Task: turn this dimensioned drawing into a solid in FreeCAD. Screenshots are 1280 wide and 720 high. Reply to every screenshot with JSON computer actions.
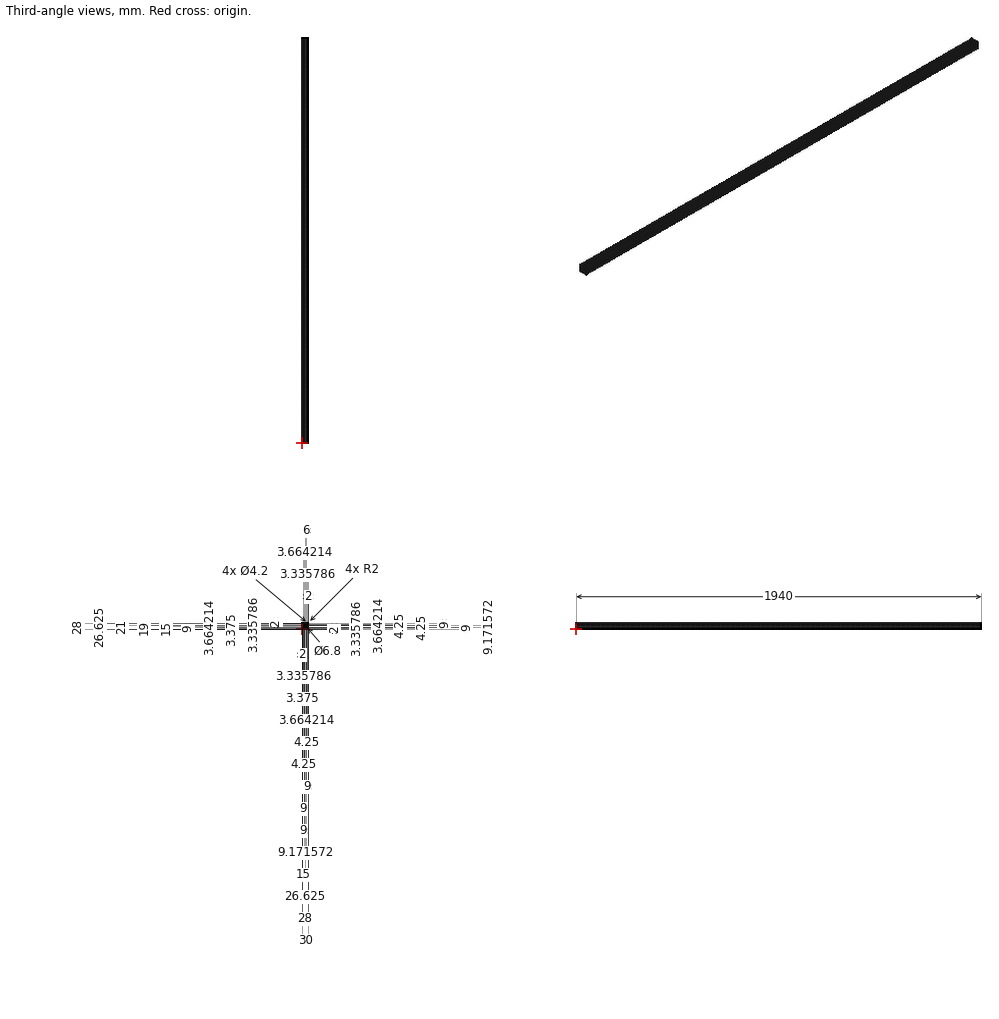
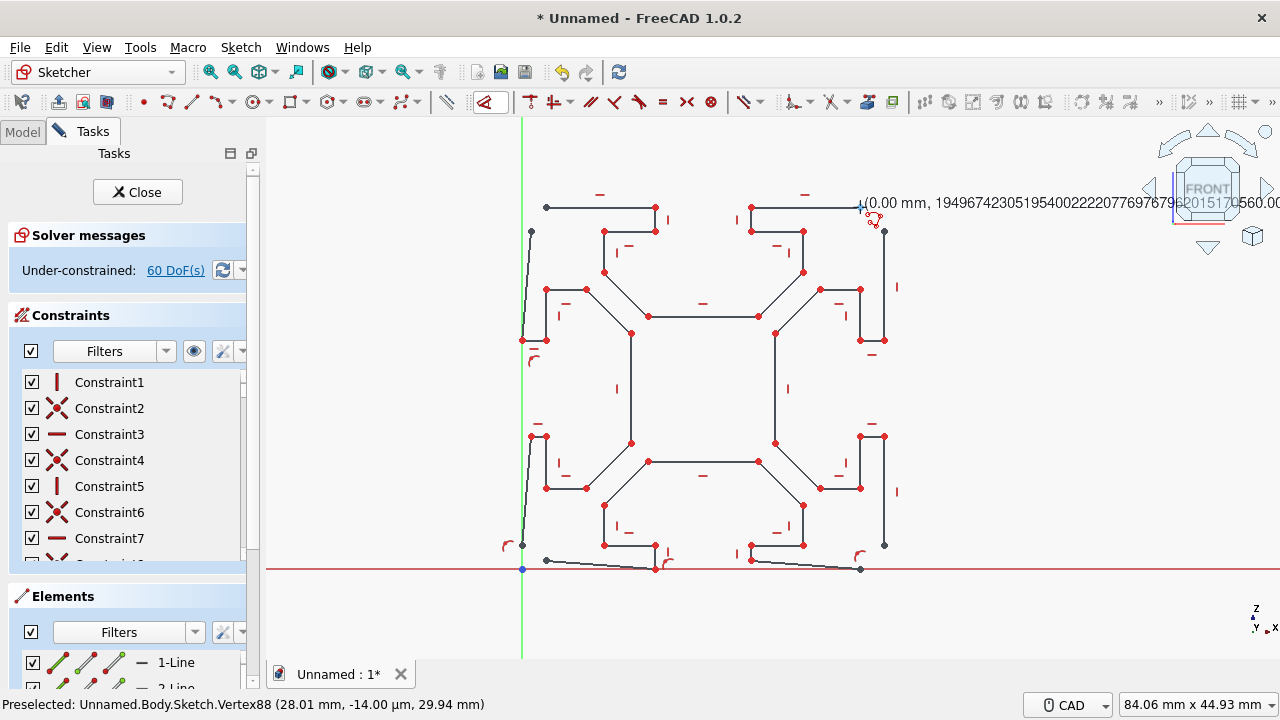
{"action": "left_click", "coordinate": [216, 102]}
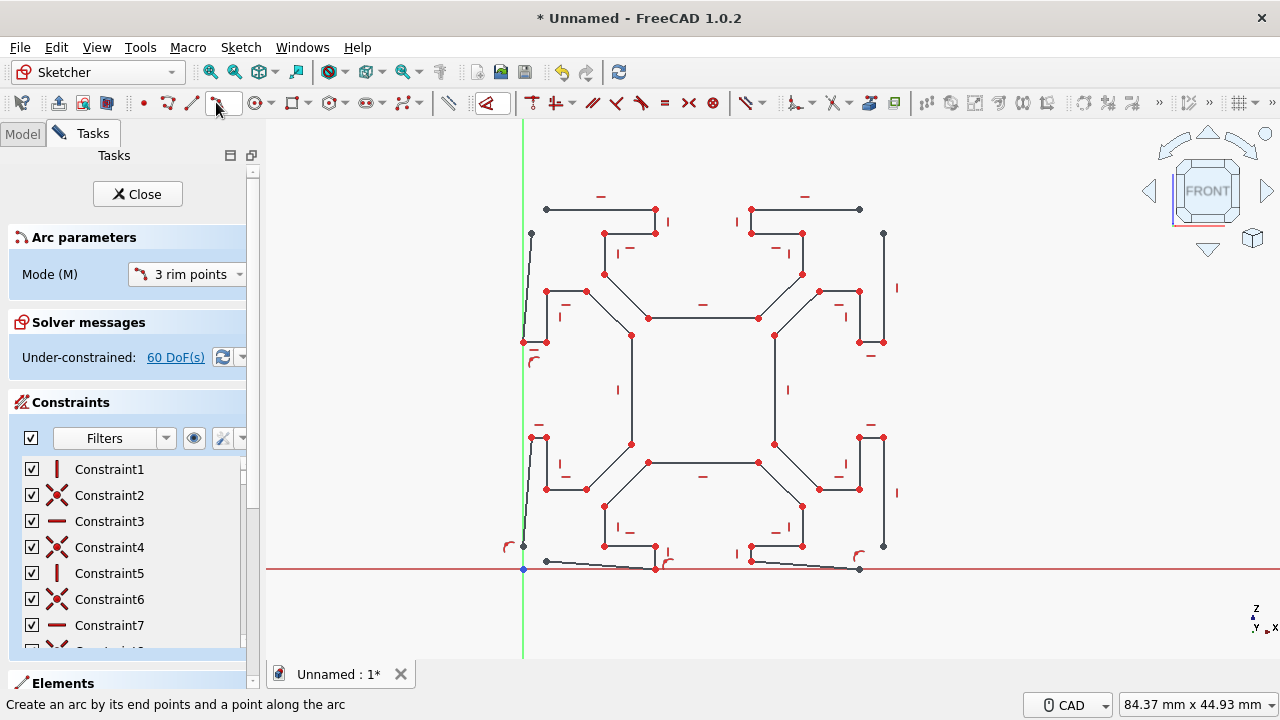
{"action": "left_click", "coordinate": [884, 546]}
{"action": "left_click", "coordinate": [860, 569]}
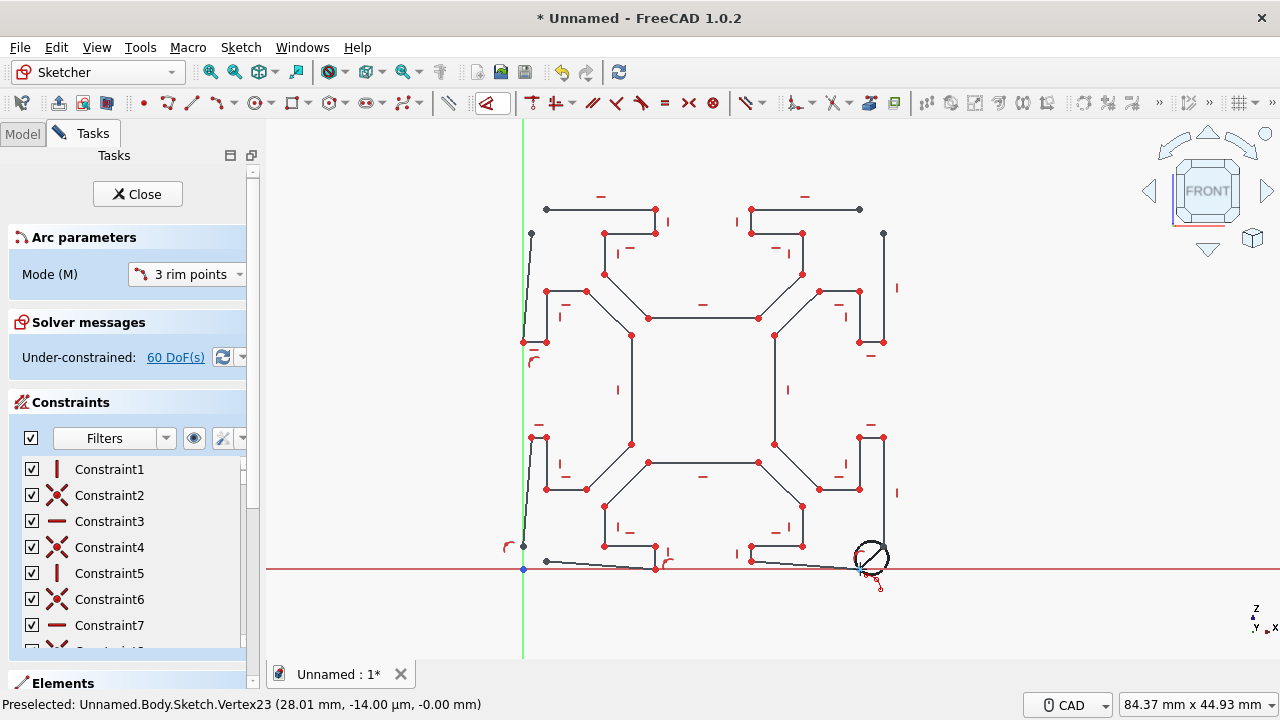
{"action": "scroll", "coordinate": [877, 562], "scroll_direction": "up", "scroll_amount": 5}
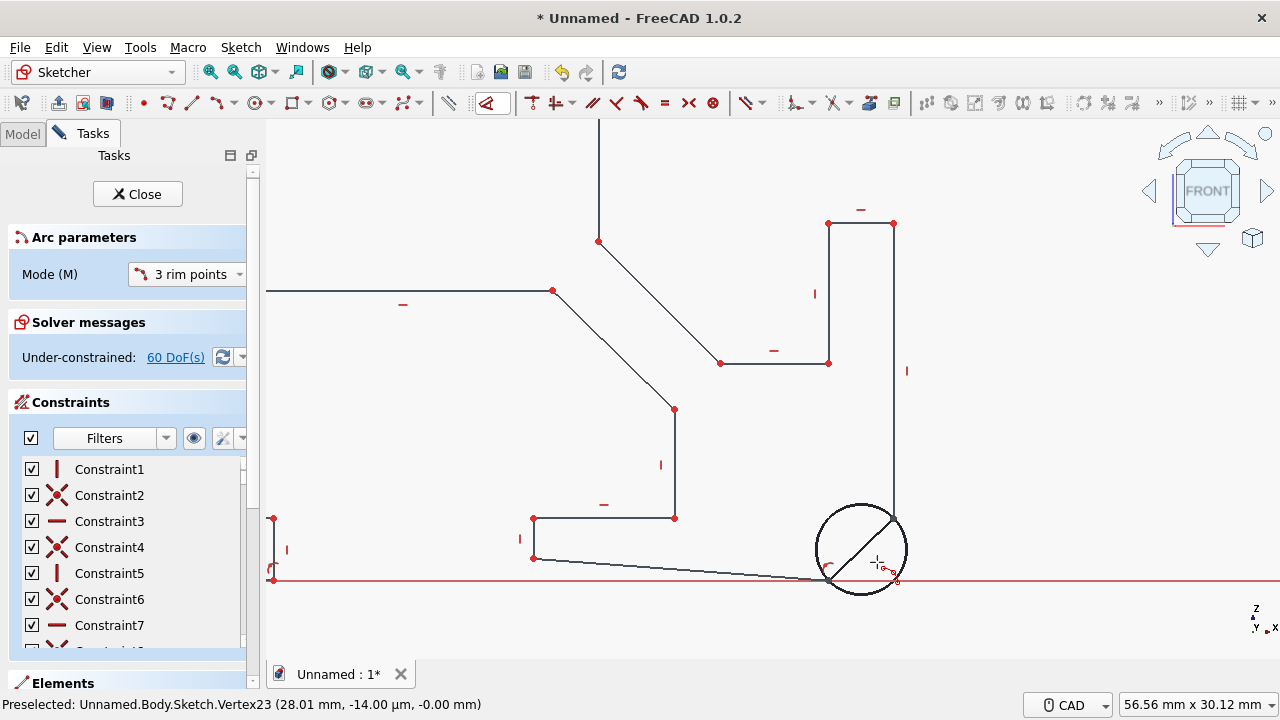
{"action": "left_click", "coordinate": [875, 562]}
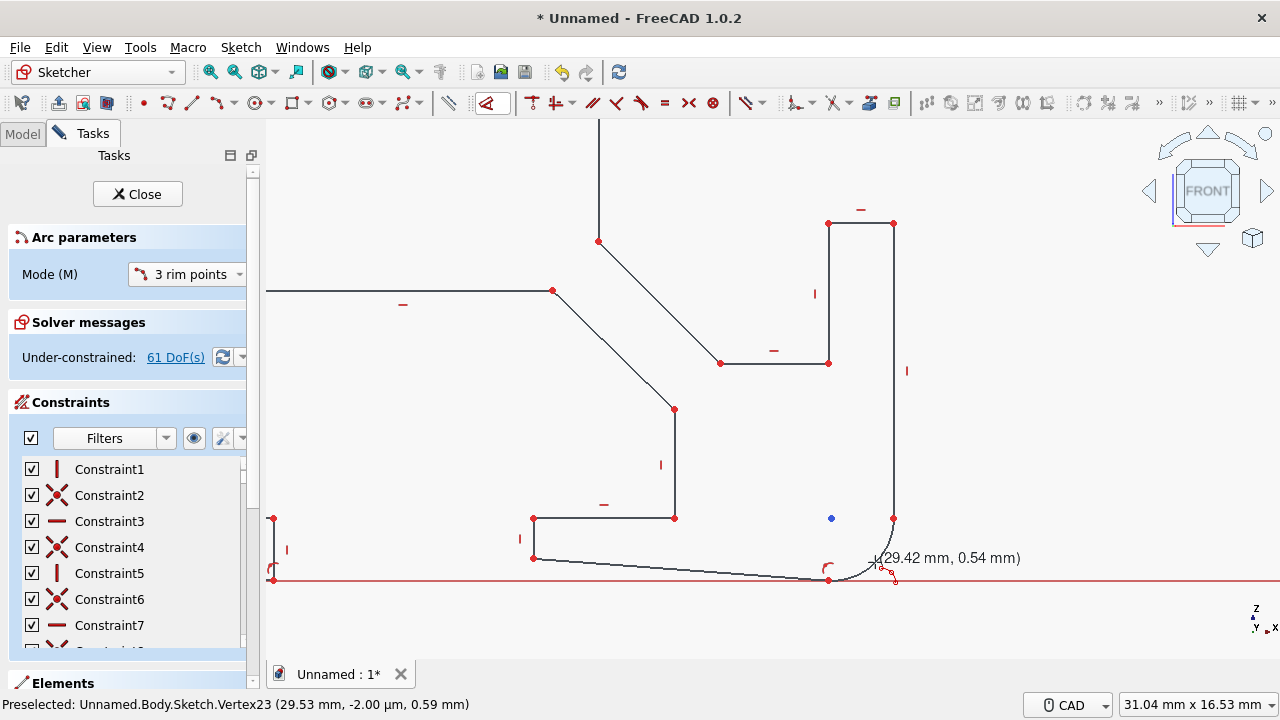
{"action": "scroll", "coordinate": [879, 563], "scroll_direction": "down", "scroll_amount": 5}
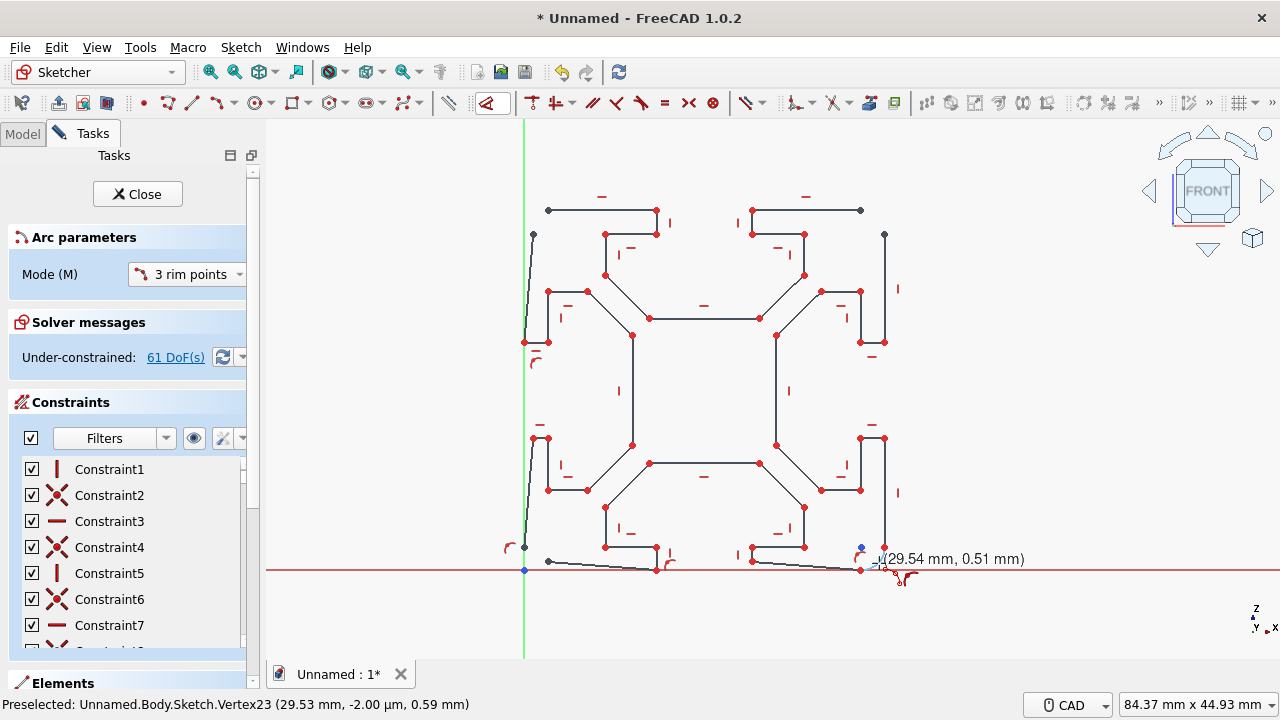
{"action": "left_click", "coordinate": [548, 562]}
{"action": "left_click", "coordinate": [524, 547]}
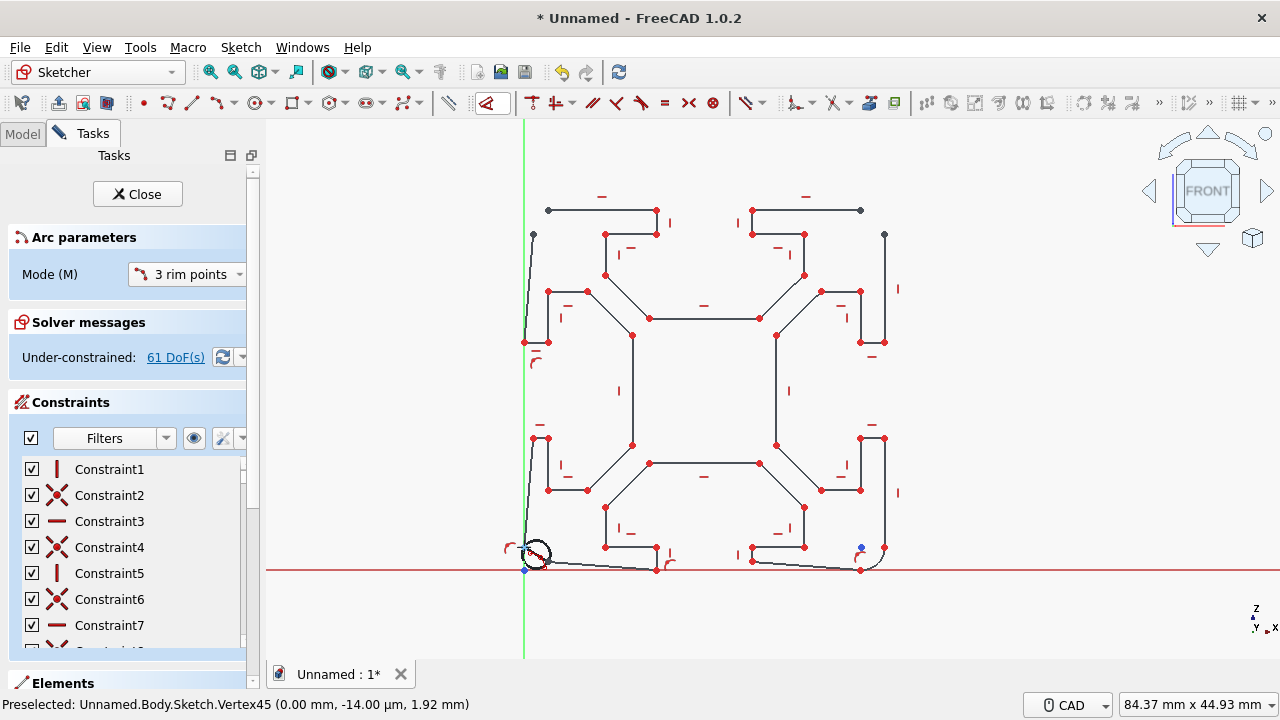
{"action": "scroll", "coordinate": [531, 563], "scroll_direction": "up", "scroll_amount": 5}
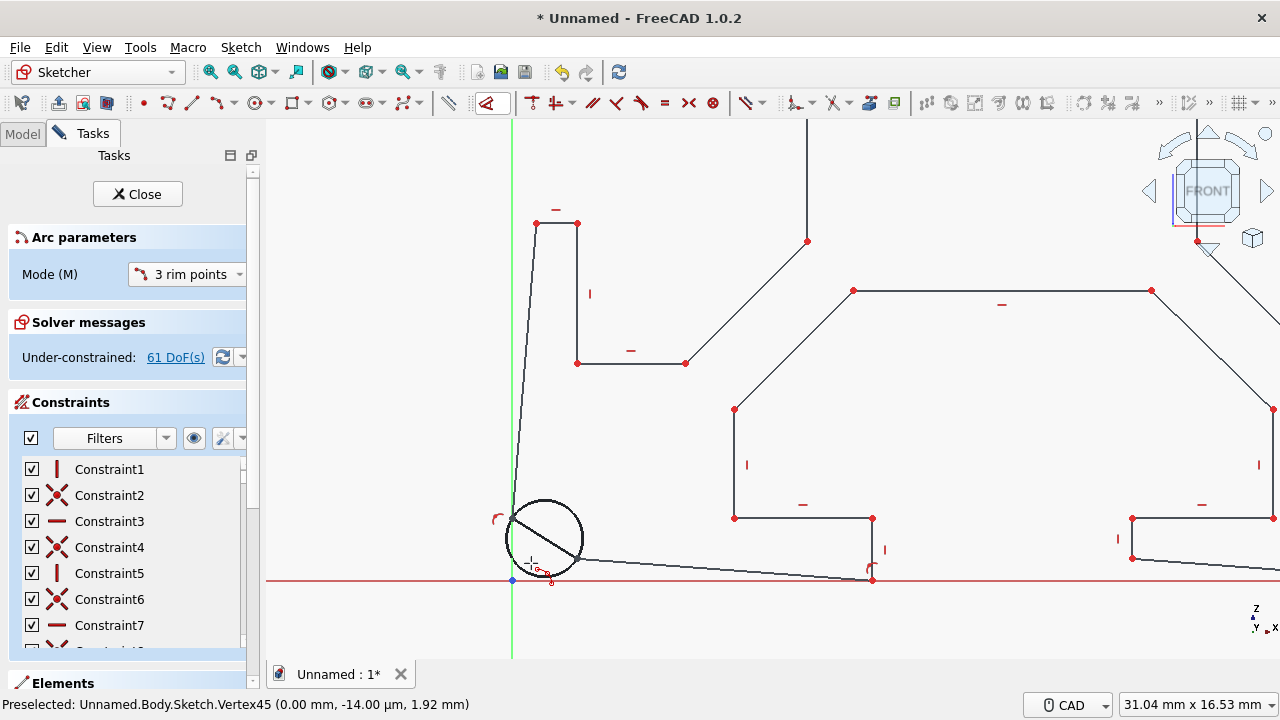
{"action": "left_click", "coordinate": [532, 562]}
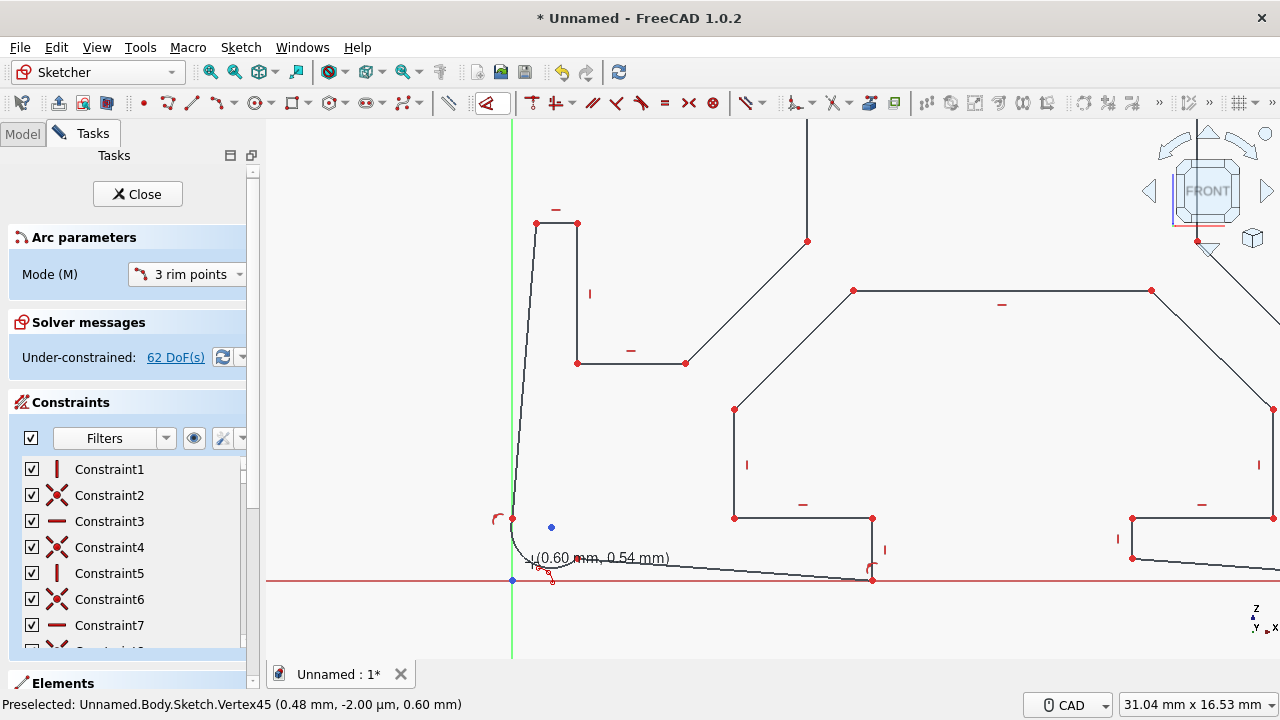
{"action": "scroll", "coordinate": [531, 563], "scroll_direction": "down", "scroll_amount": 5}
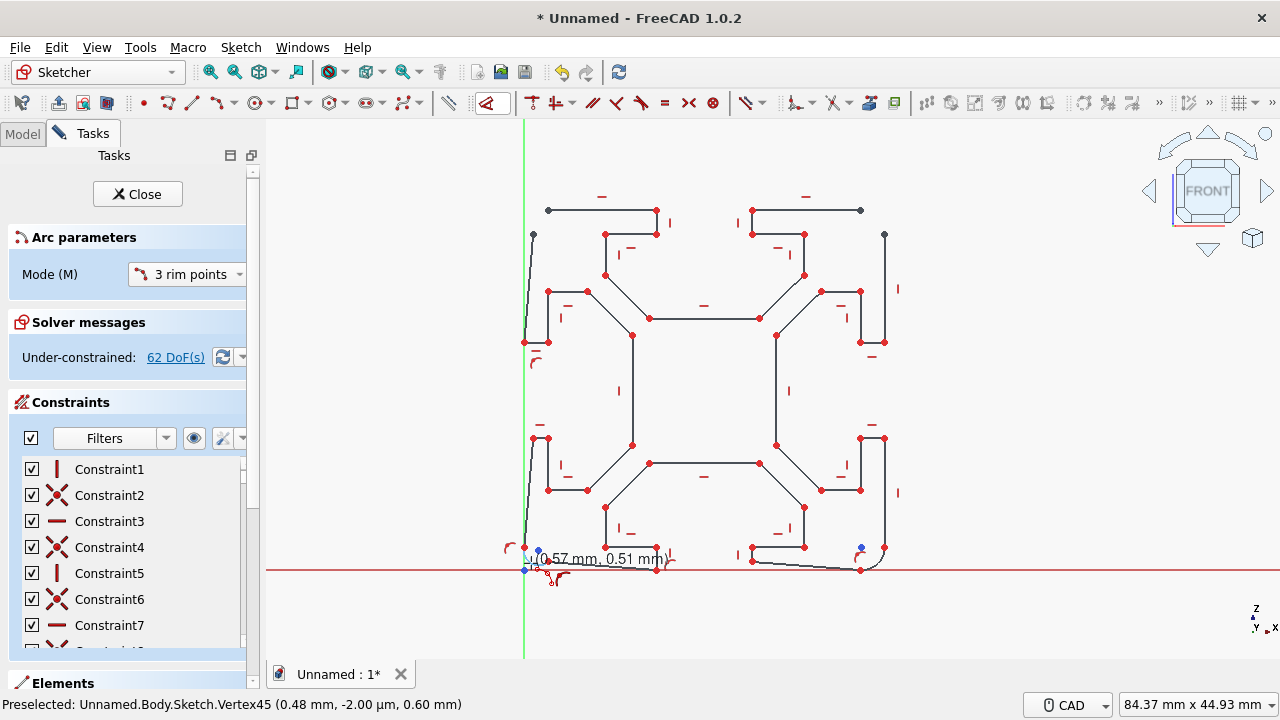
{"action": "left_click", "coordinate": [533, 234]}
{"action": "left_click", "coordinate": [548, 210]}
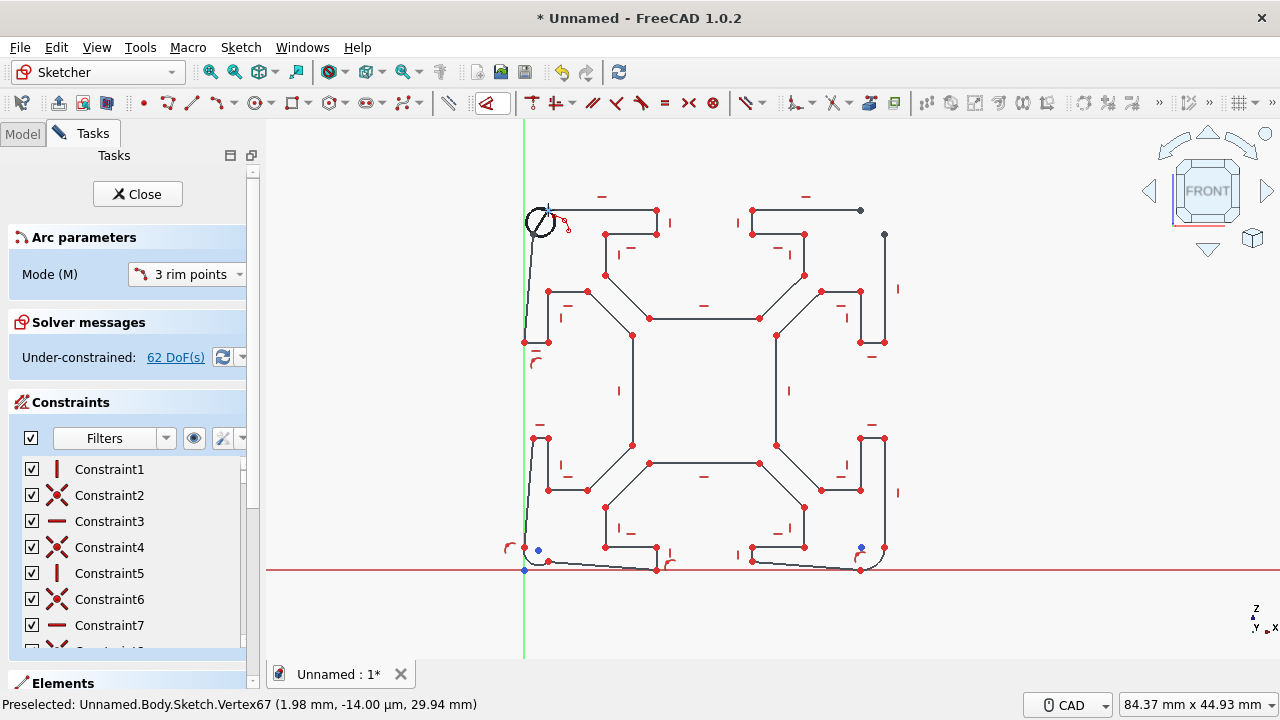
{"action": "scroll", "coordinate": [531, 217], "scroll_direction": "up", "scroll_amount": 5}